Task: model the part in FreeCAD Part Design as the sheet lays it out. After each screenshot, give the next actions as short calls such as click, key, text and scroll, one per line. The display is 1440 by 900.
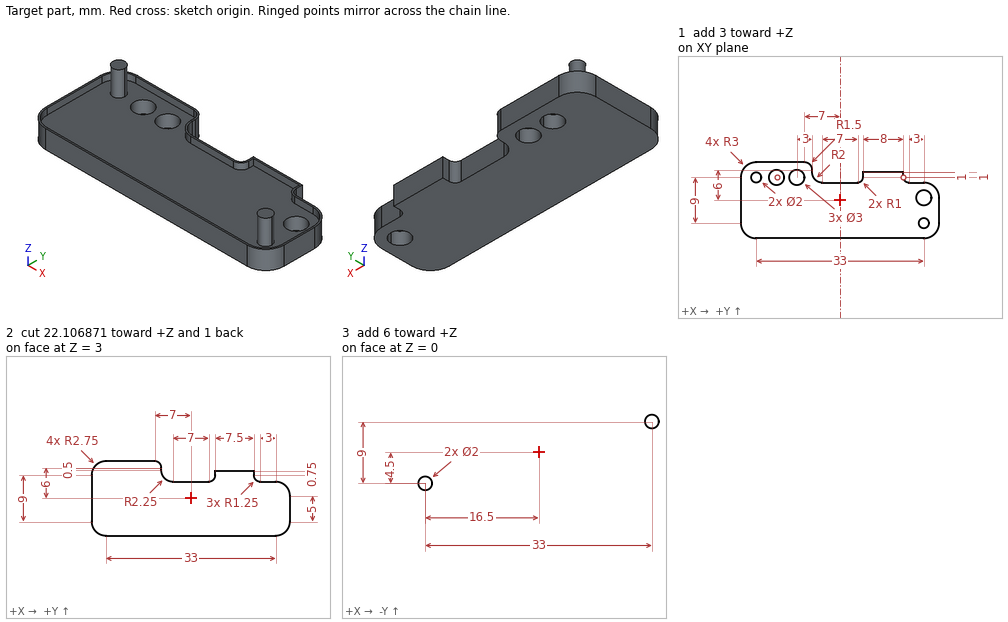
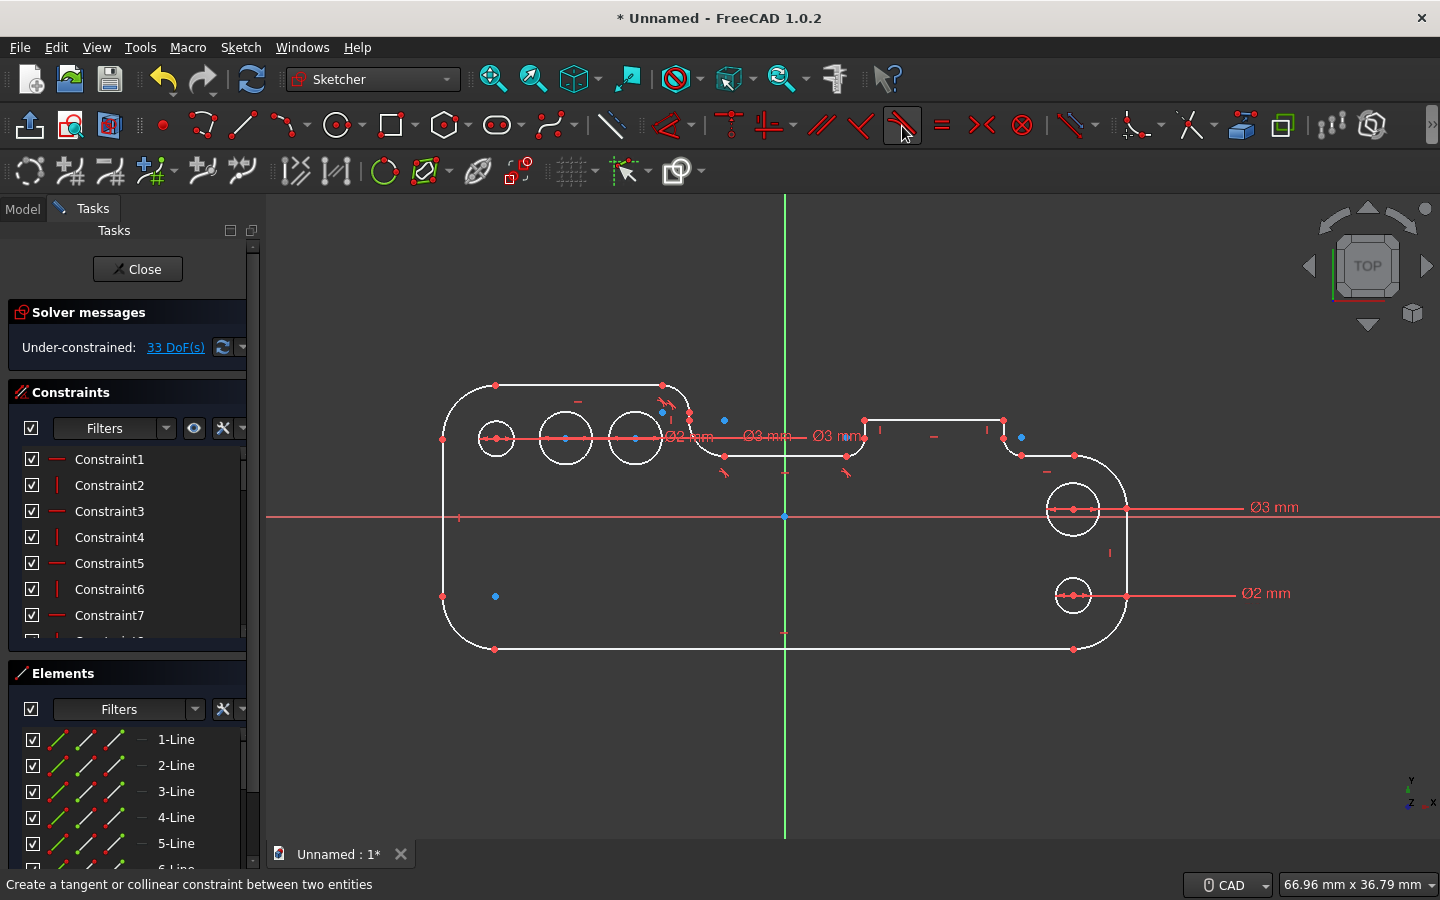
click(612, 385)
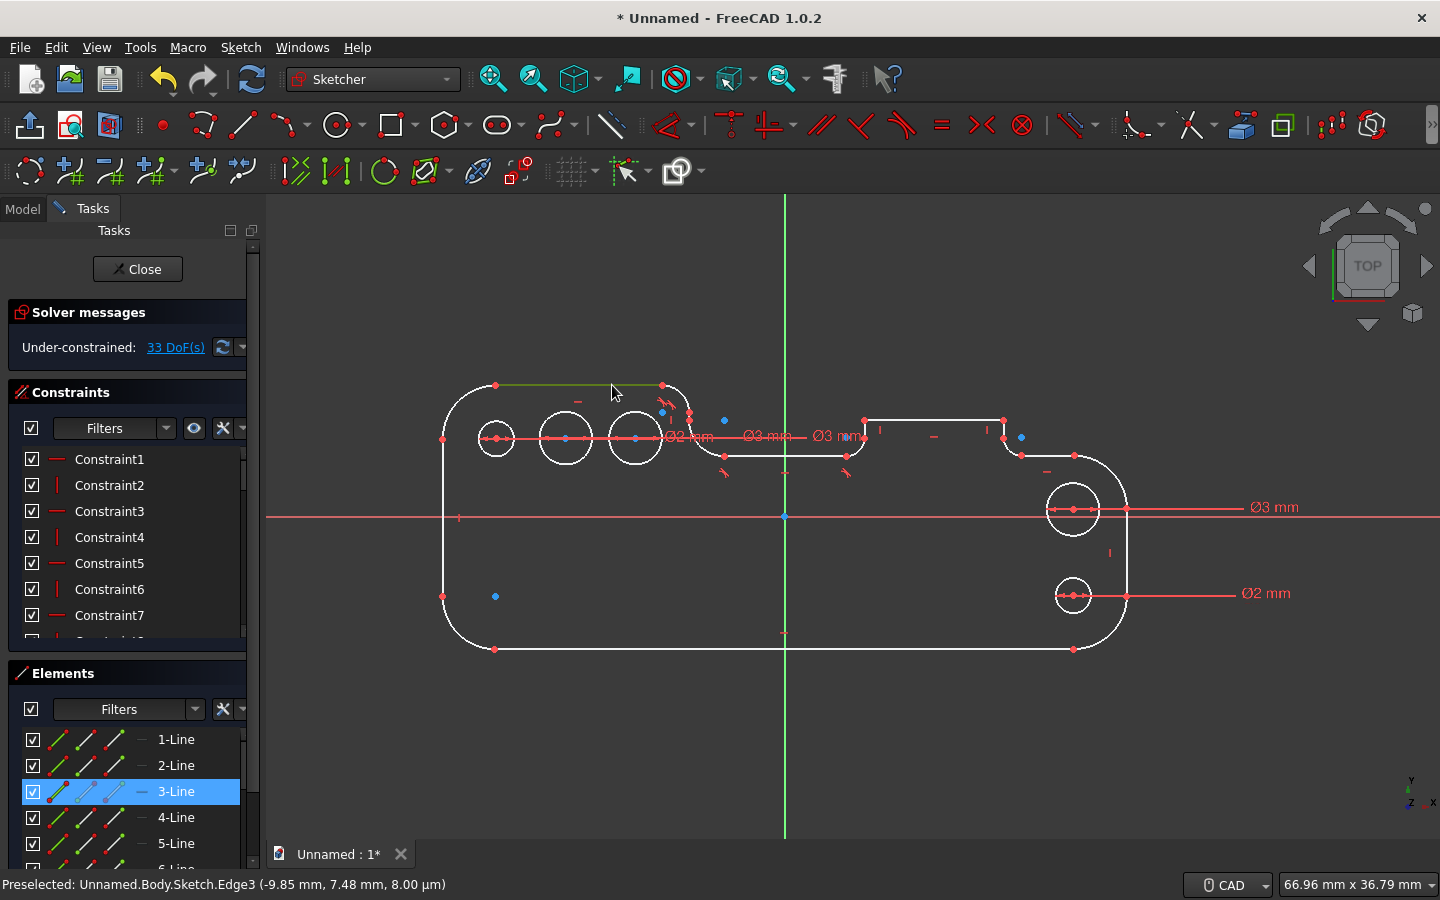
click(471, 392)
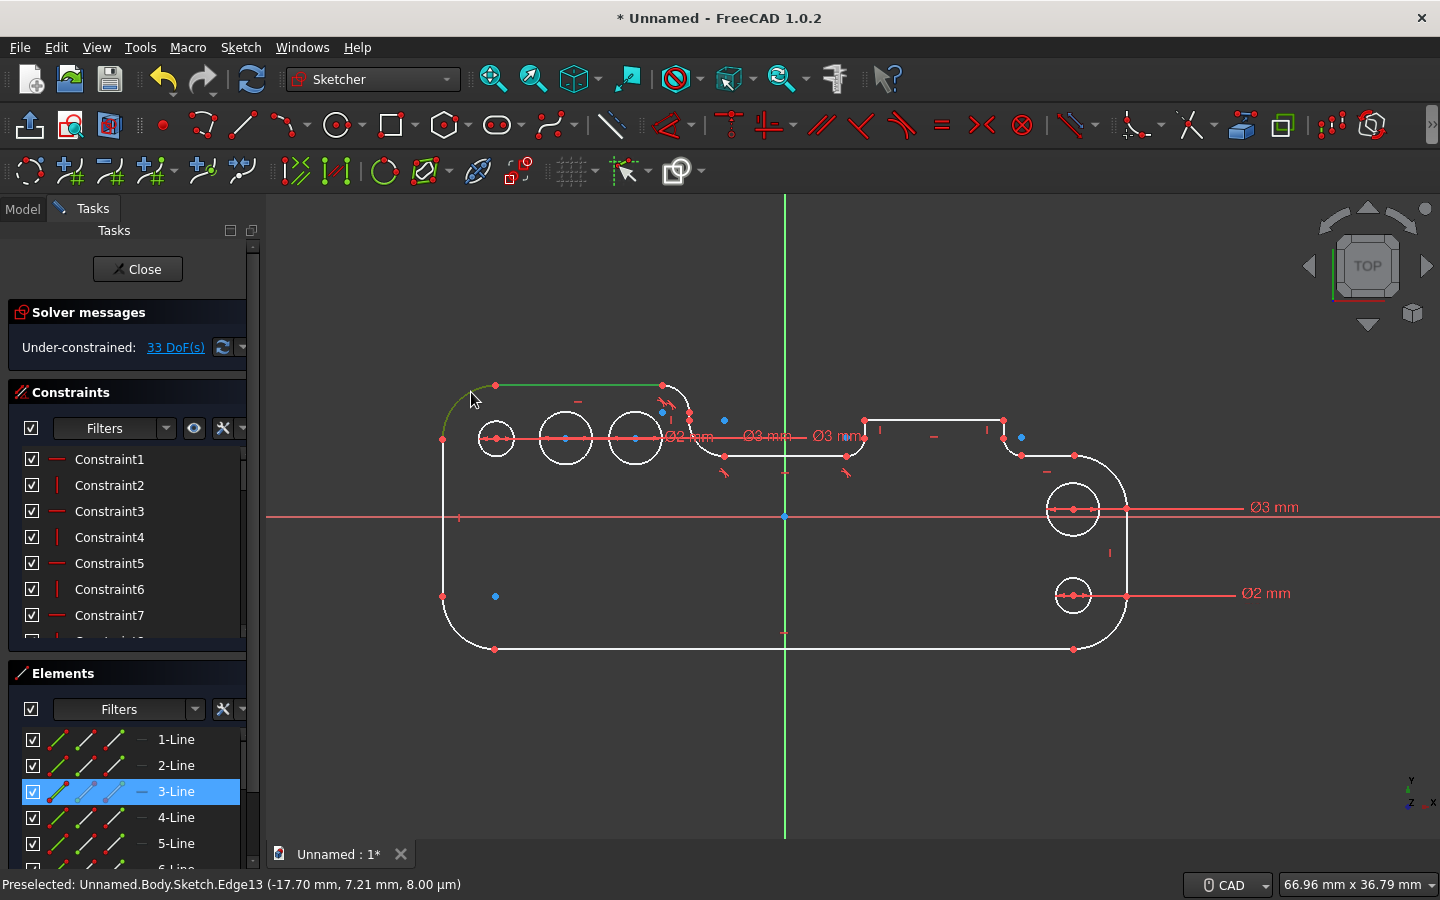
click(902, 126)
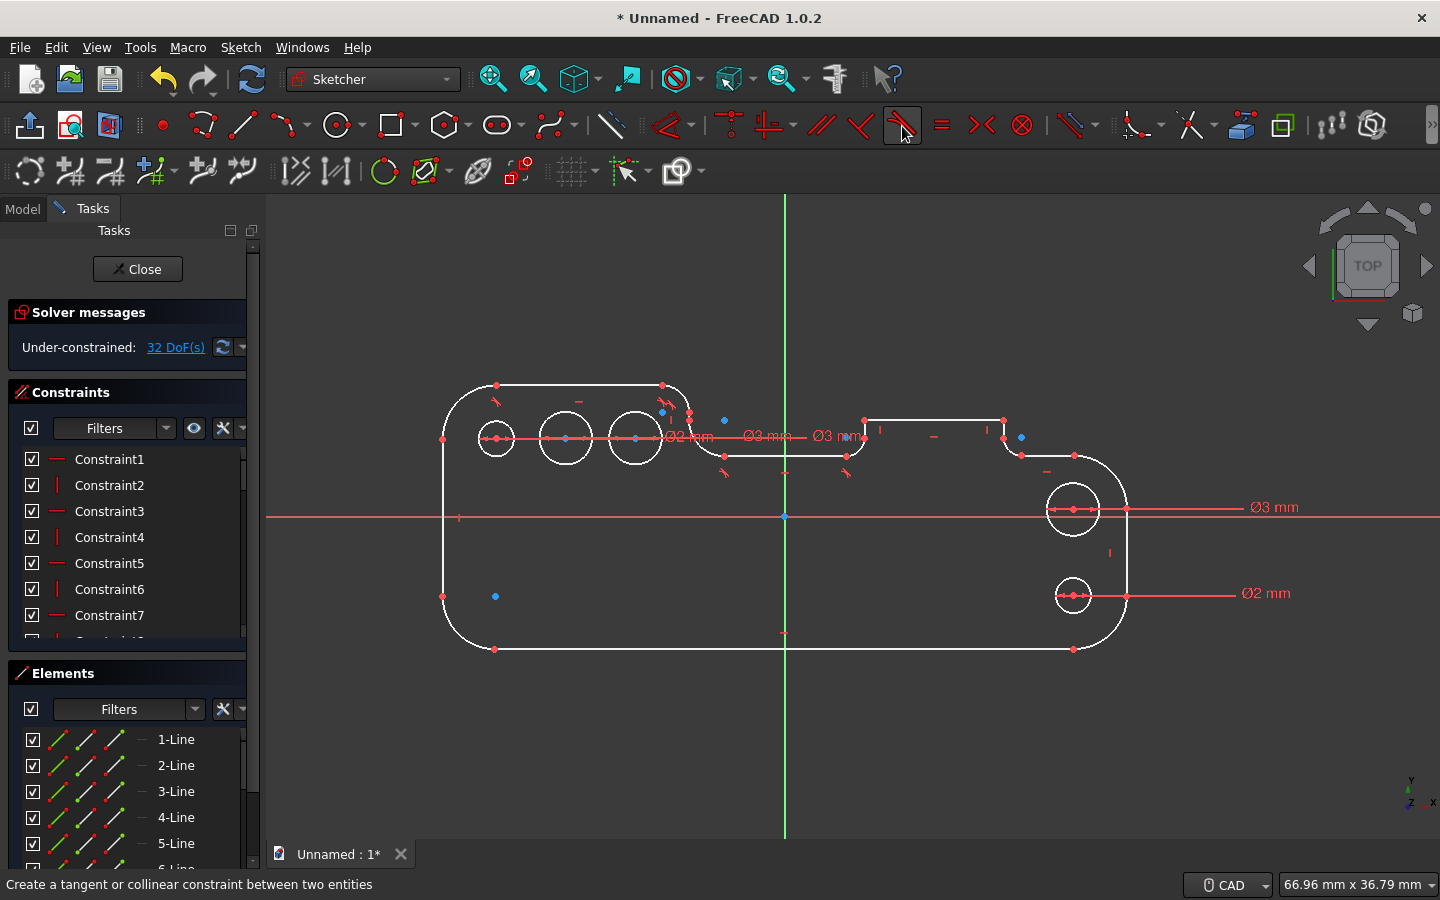
click(443, 486)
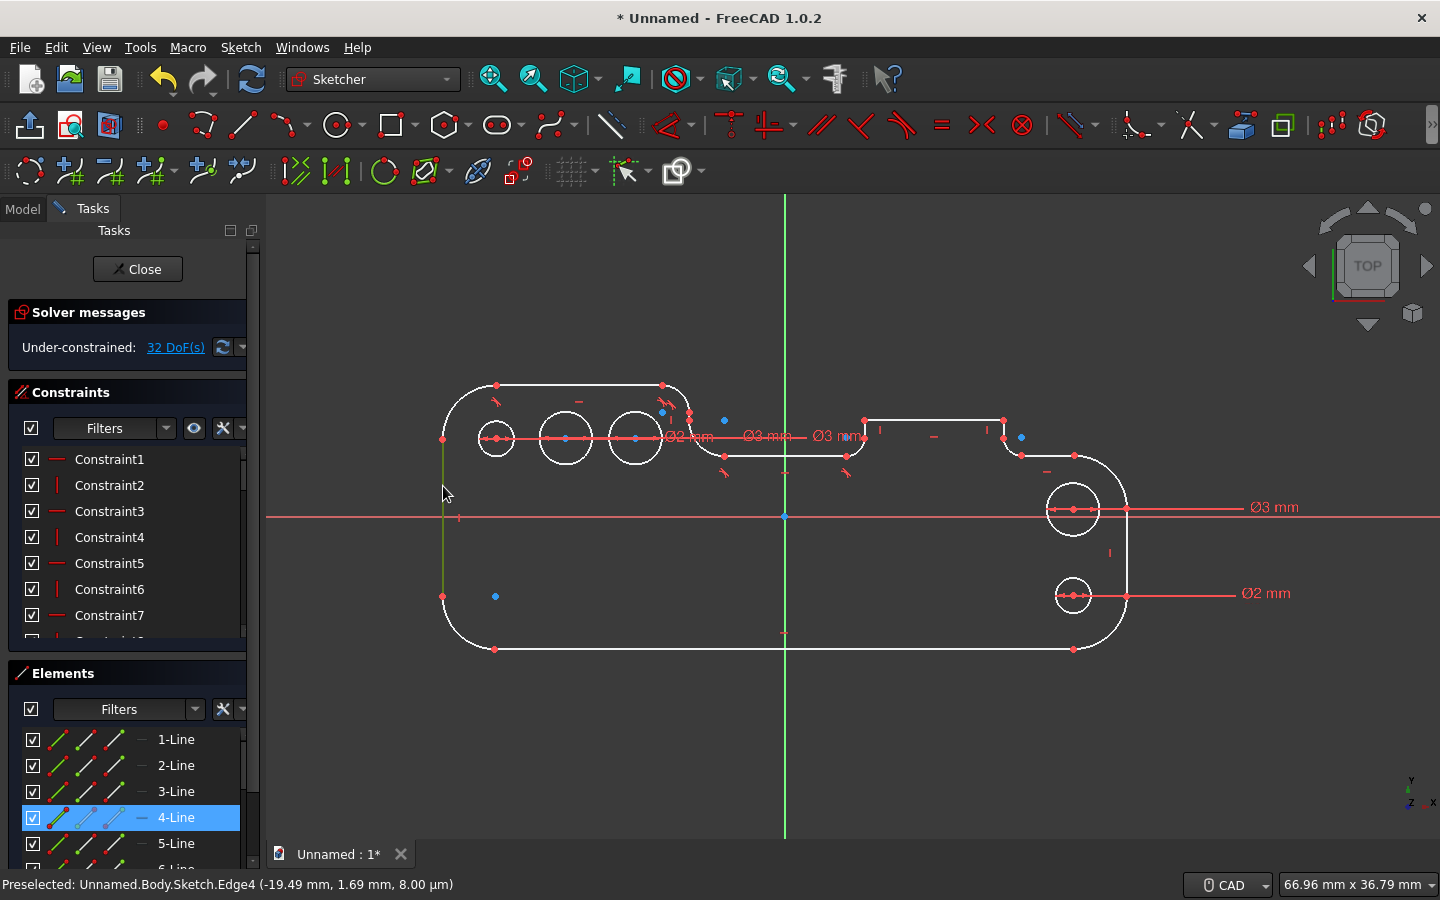
click(472, 391)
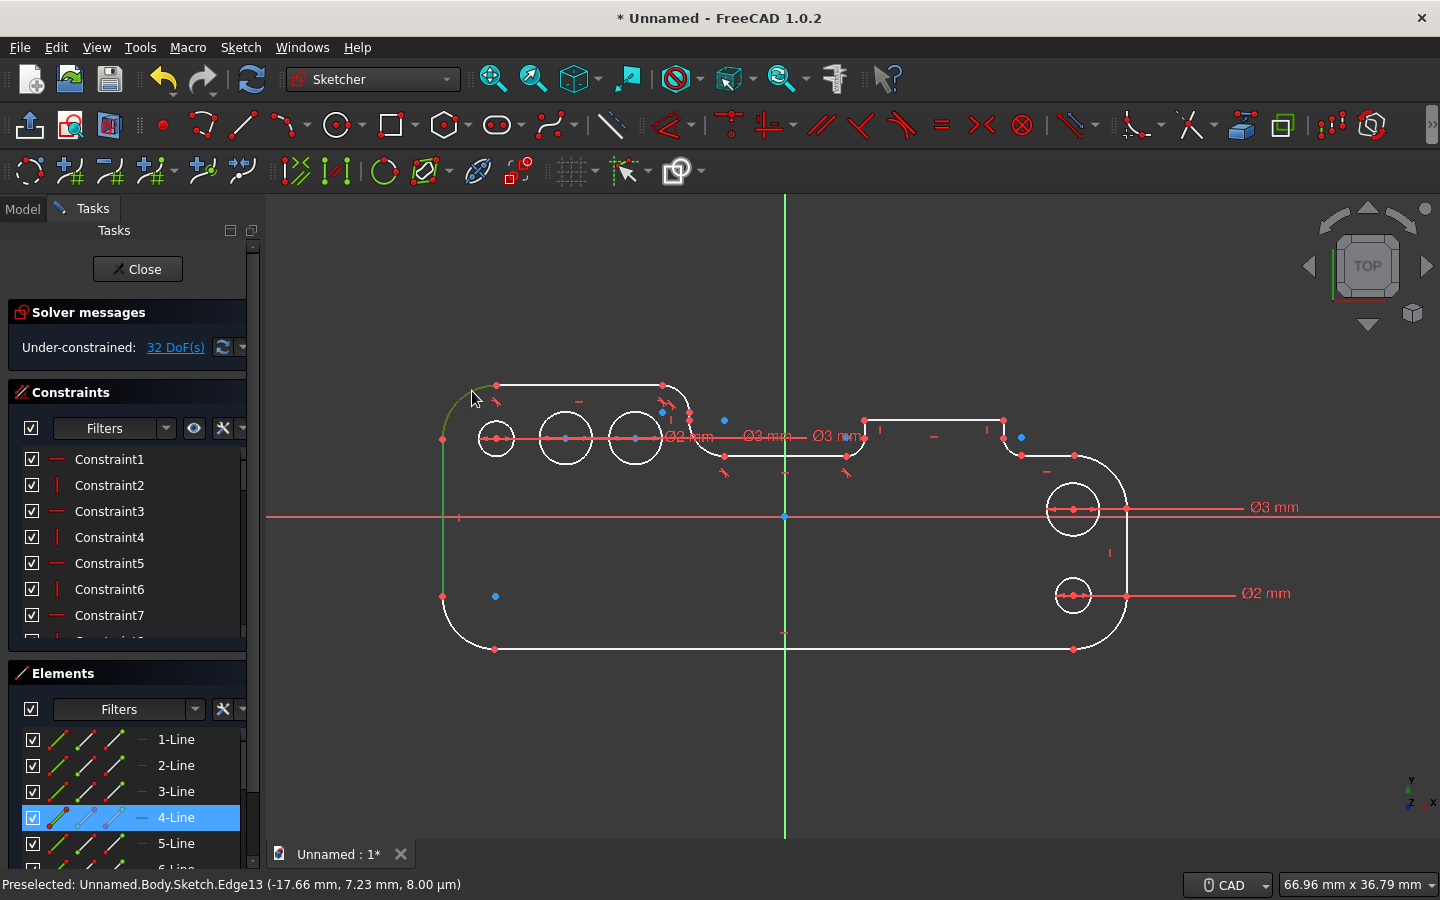
key(t)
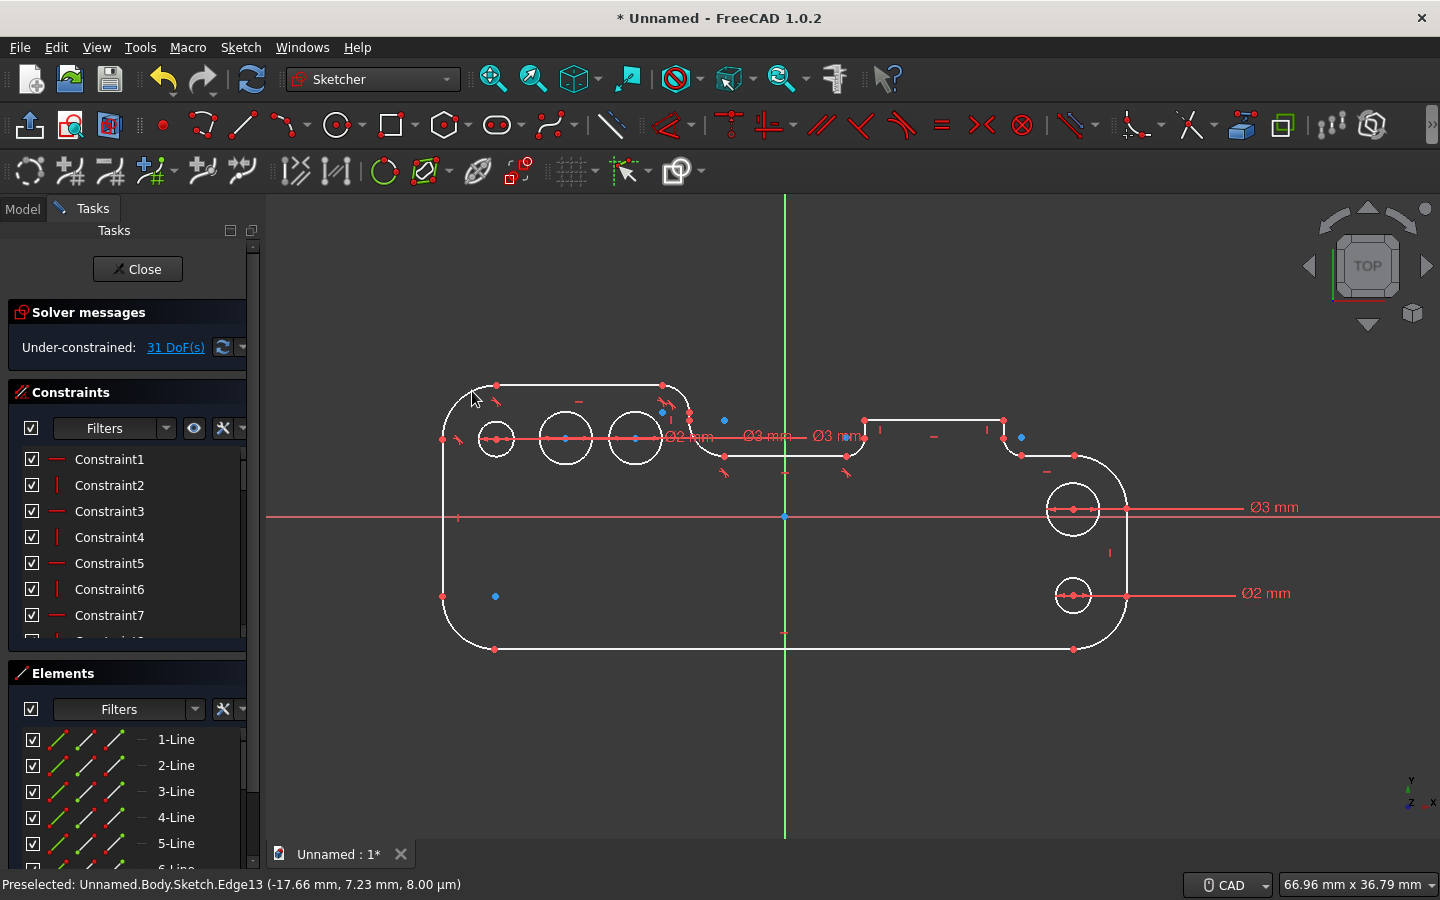
click(443, 486)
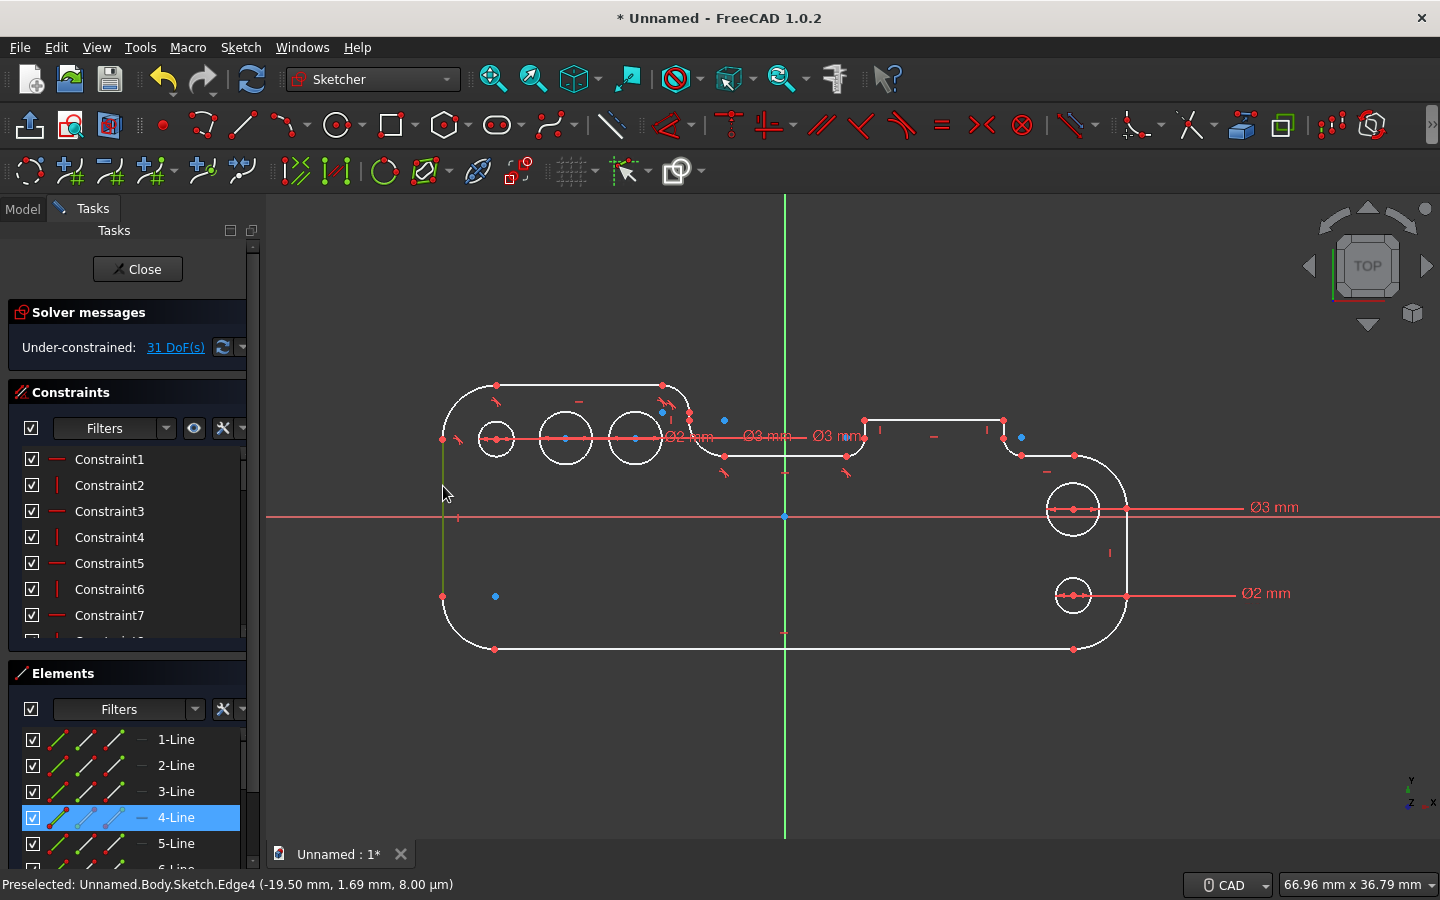
click(448, 620)